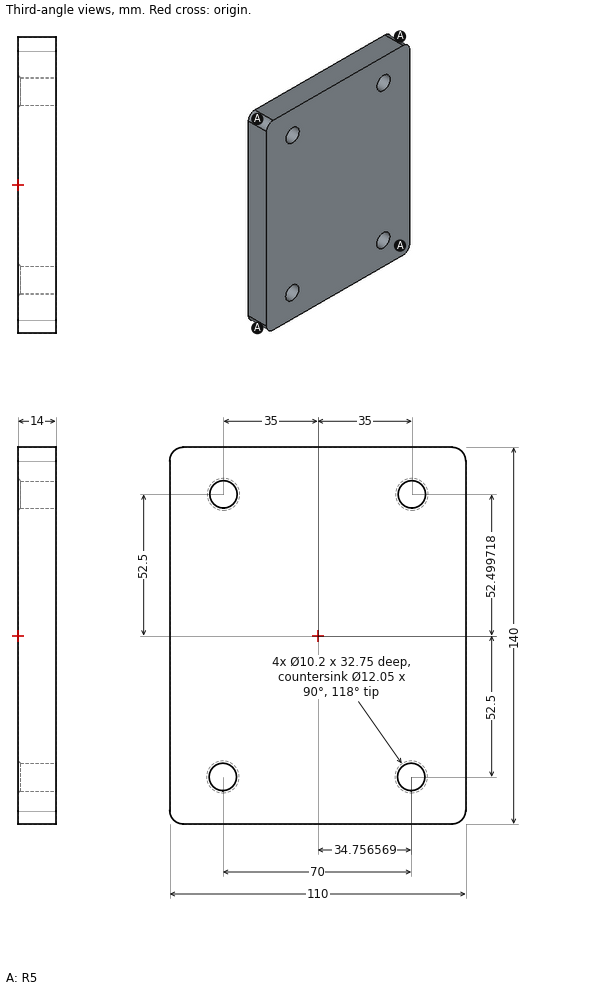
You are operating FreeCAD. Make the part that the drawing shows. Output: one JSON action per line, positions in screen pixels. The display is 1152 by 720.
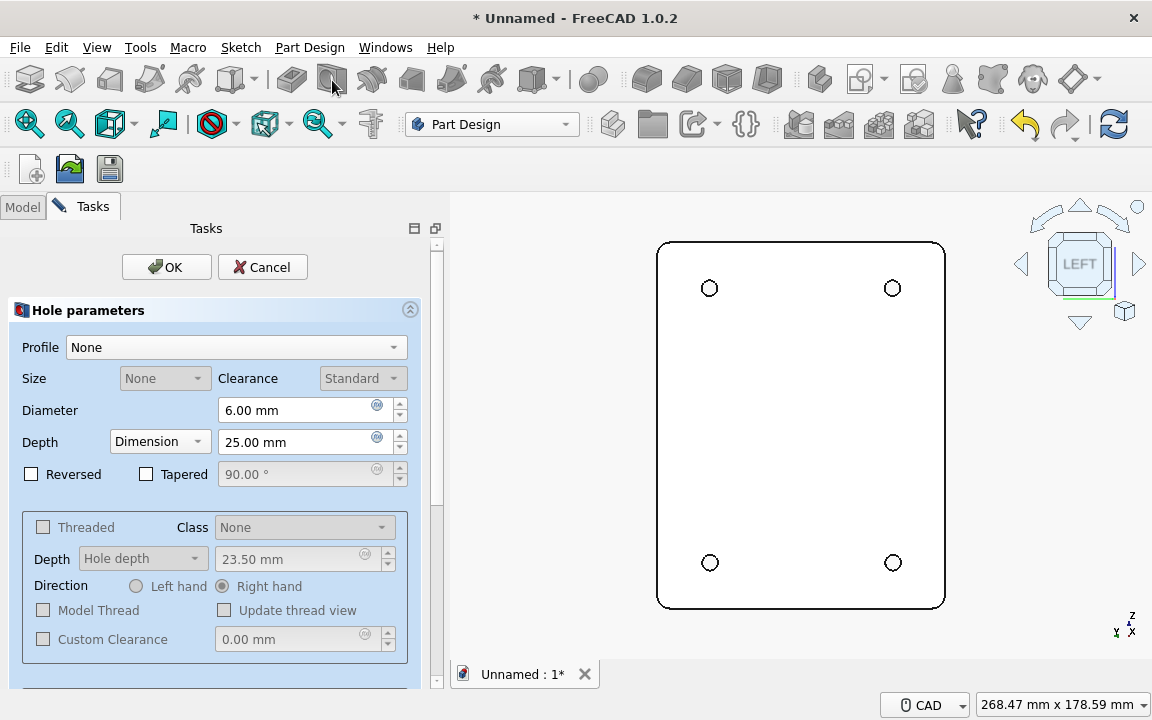
{"action": "triple_click", "coordinate": [305, 410]}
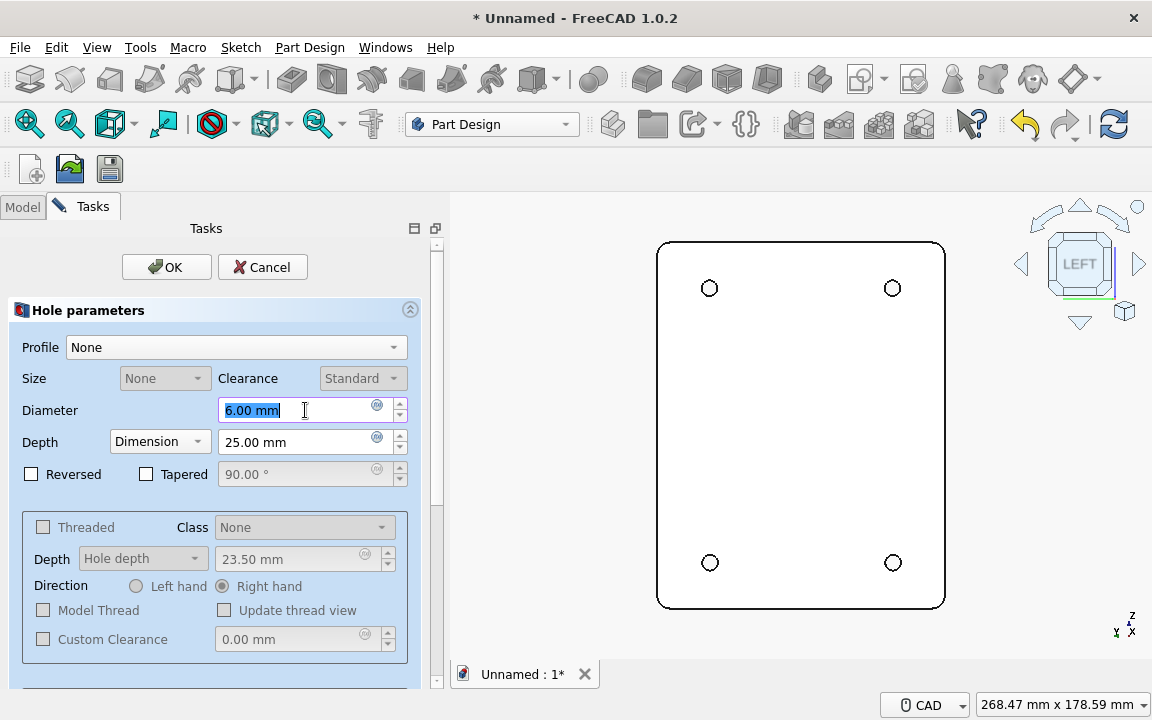
{"action": "type", "text": "10.2"}
{"action": "key", "text": "Tab"}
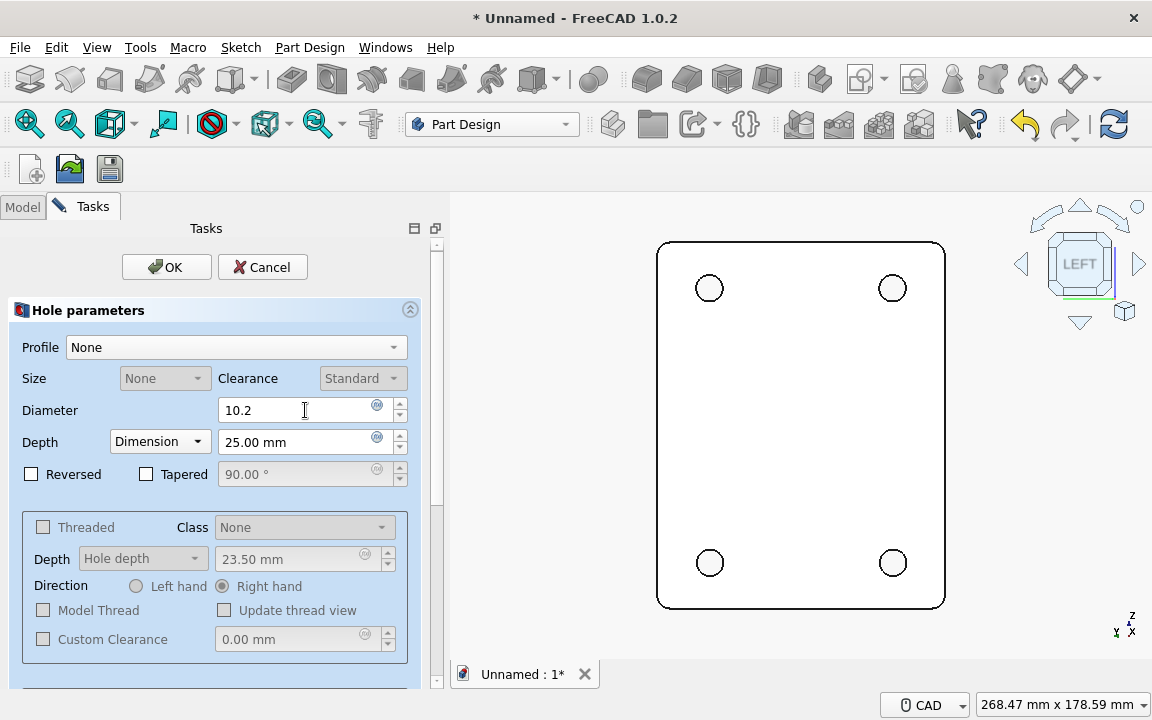
{"action": "triple_click", "coordinate": [305, 442]}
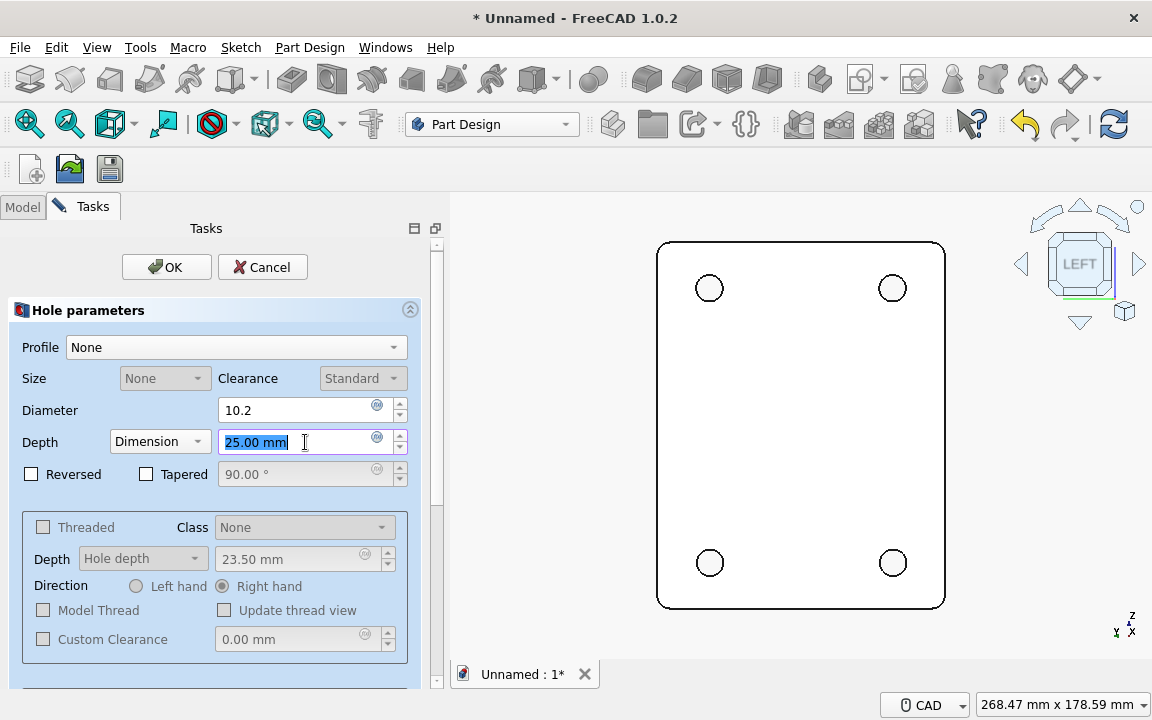
{"action": "type", "text": "32.75"}
{"action": "key", "text": "Tab"}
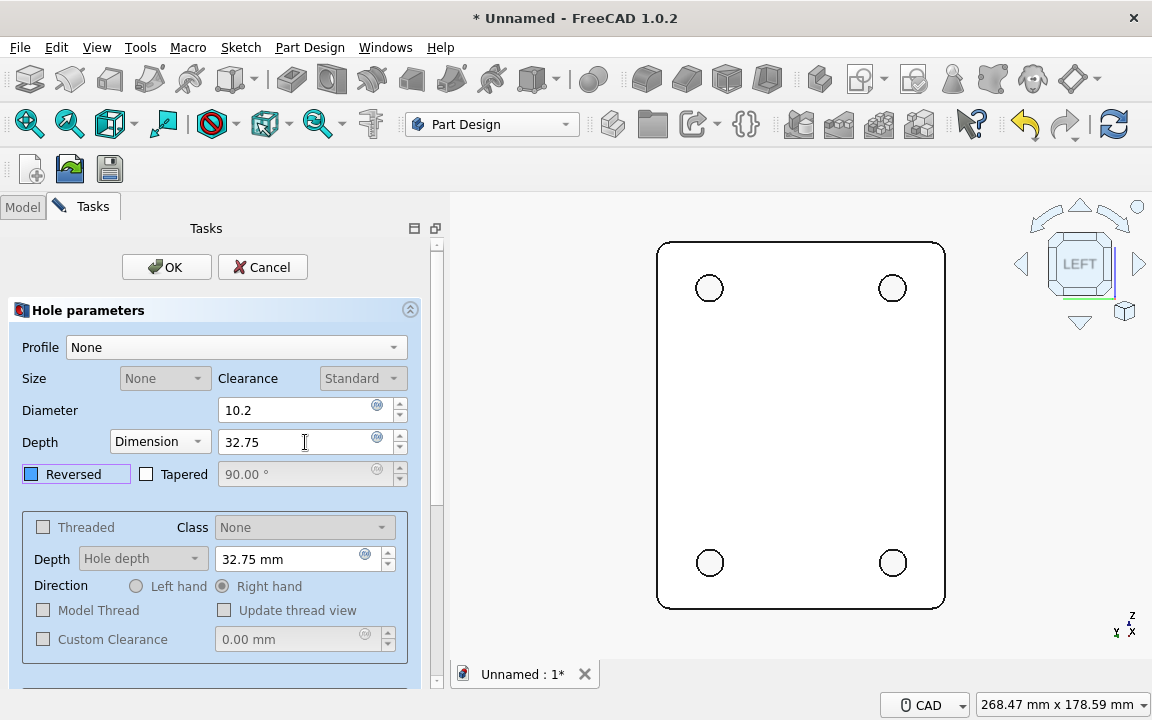
{"action": "scroll", "coordinate": [437, 463], "scroll_direction": "down", "scroll_amount": 2}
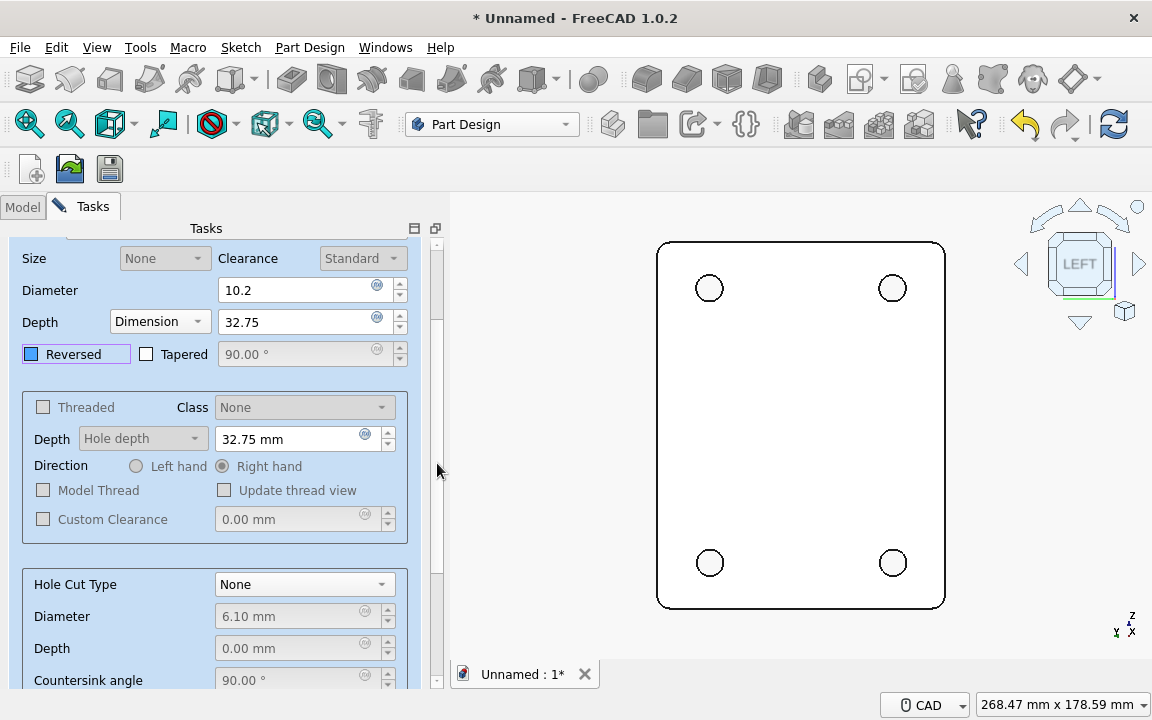
{"action": "left_click", "coordinate": [306, 584]}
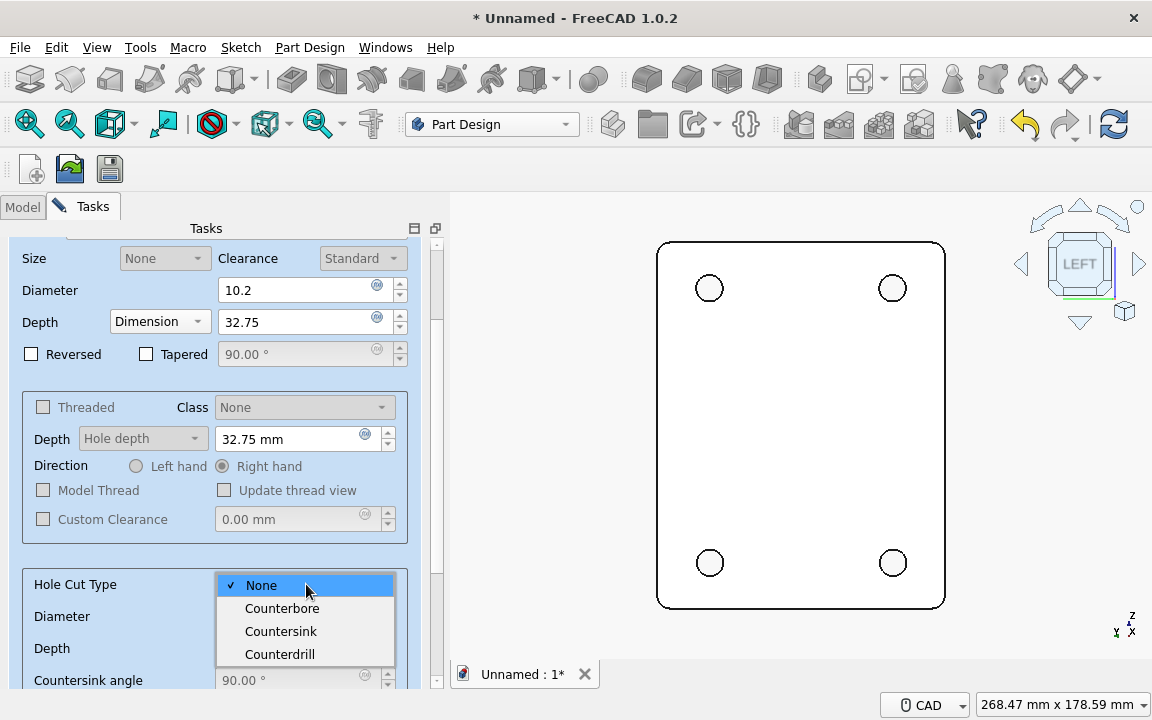
{"action": "left_click", "coordinate": [304, 632]}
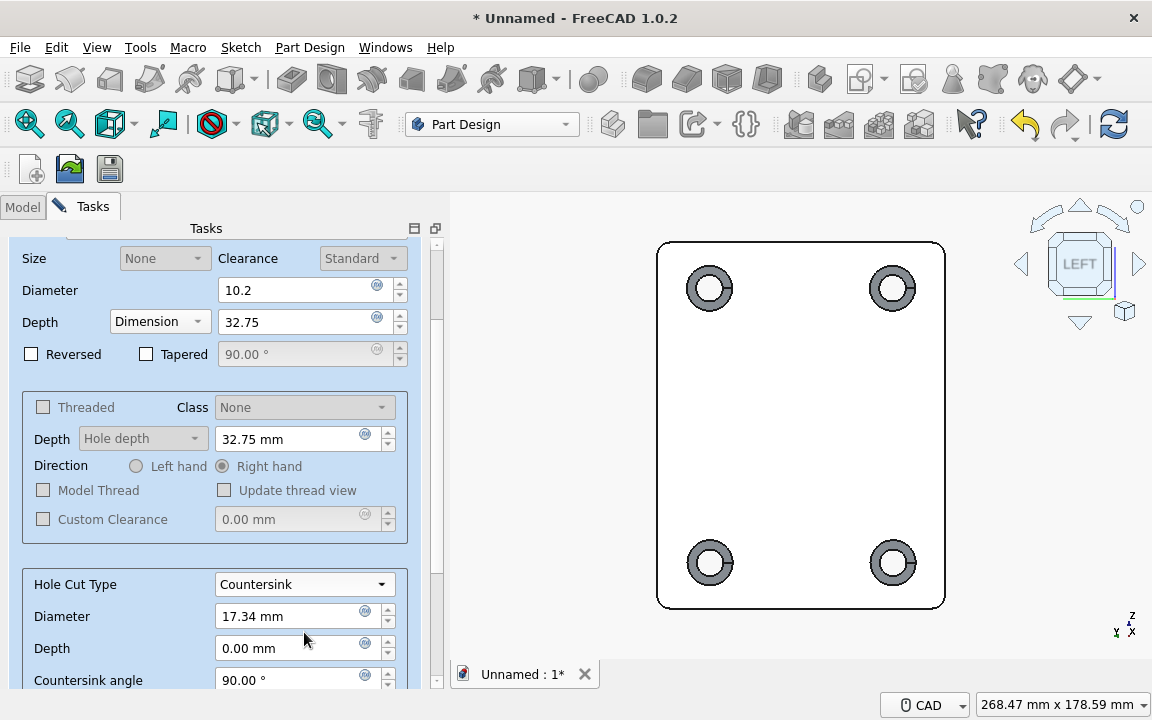
{"action": "triple_click", "coordinate": [298, 616]}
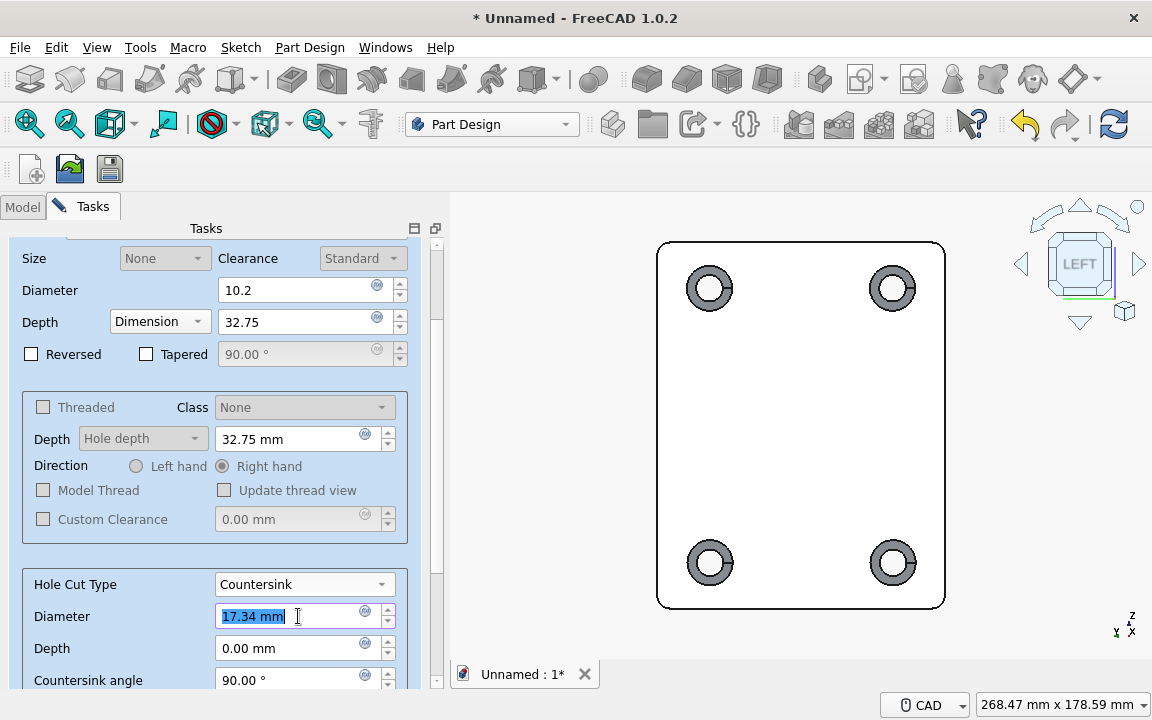
{"action": "type", "text": "12.05"}
{"action": "key", "text": "Tab"}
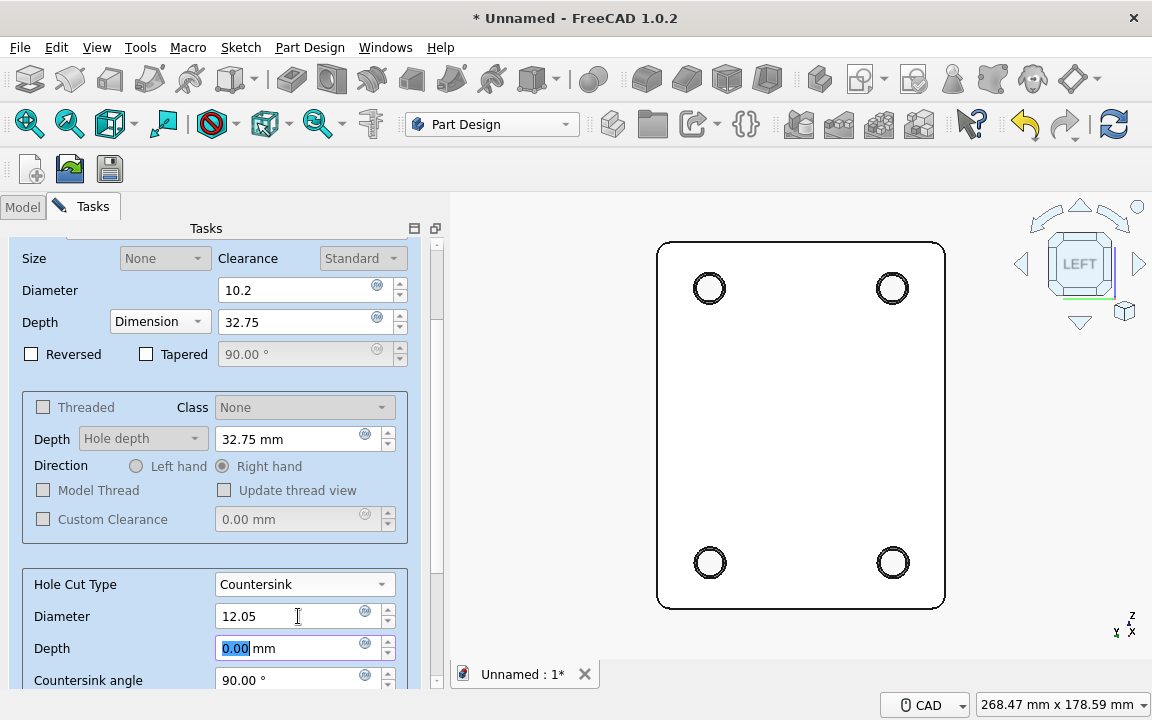
{"action": "scroll", "coordinate": [437, 463], "scroll_direction": "up", "scroll_amount": 3}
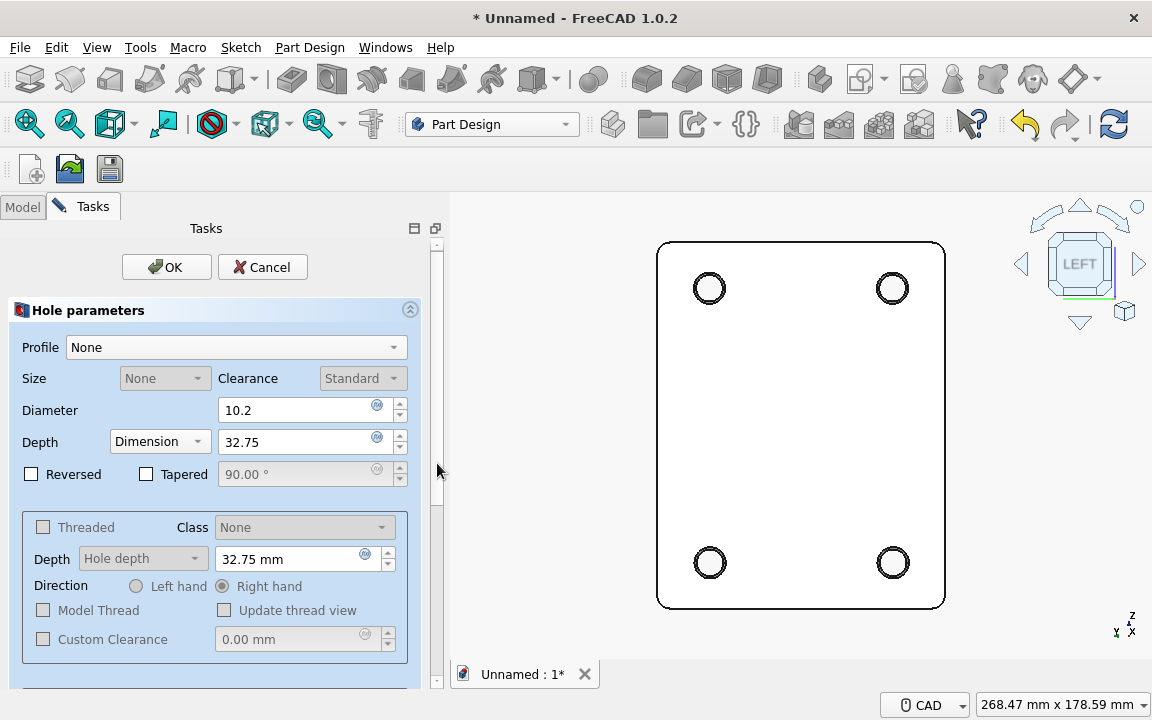
{"action": "left_click", "coordinate": [167, 267]}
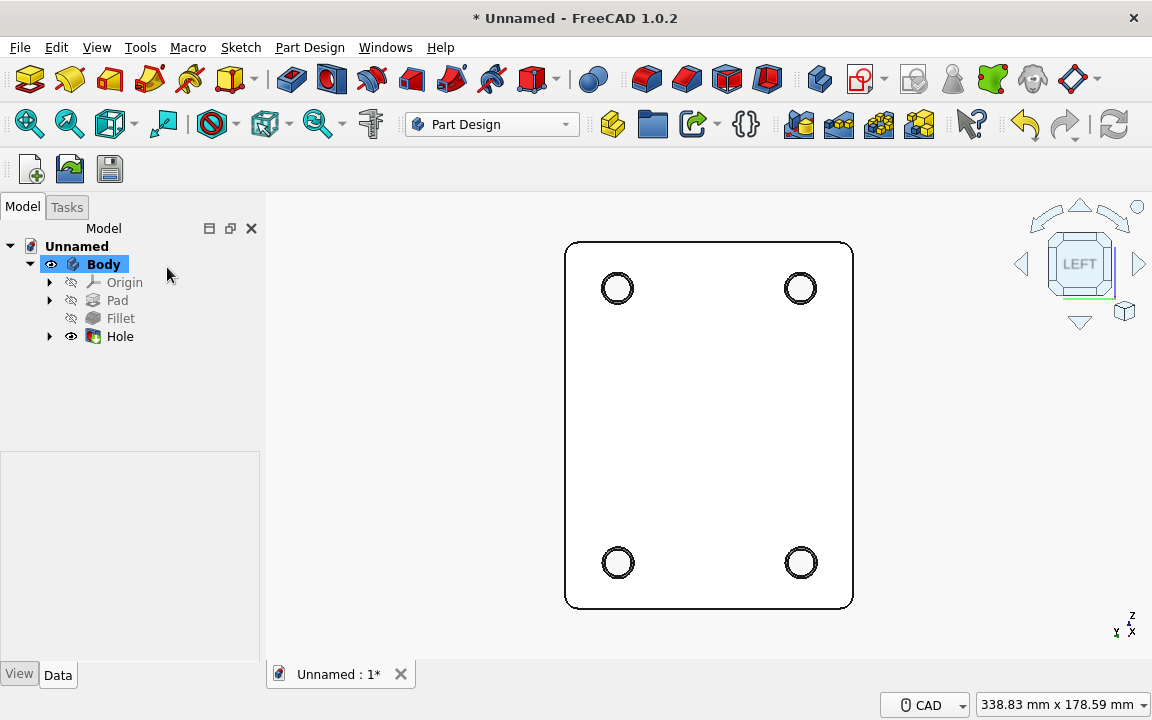
{"action": "key", "text": "0"}